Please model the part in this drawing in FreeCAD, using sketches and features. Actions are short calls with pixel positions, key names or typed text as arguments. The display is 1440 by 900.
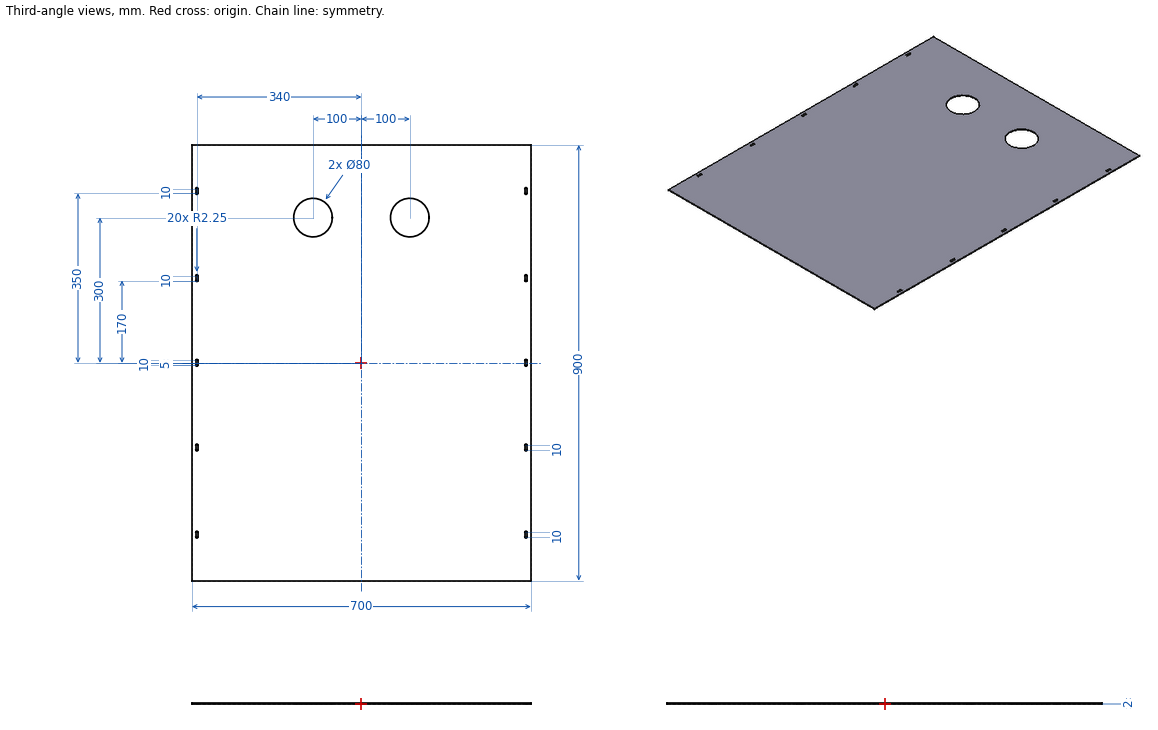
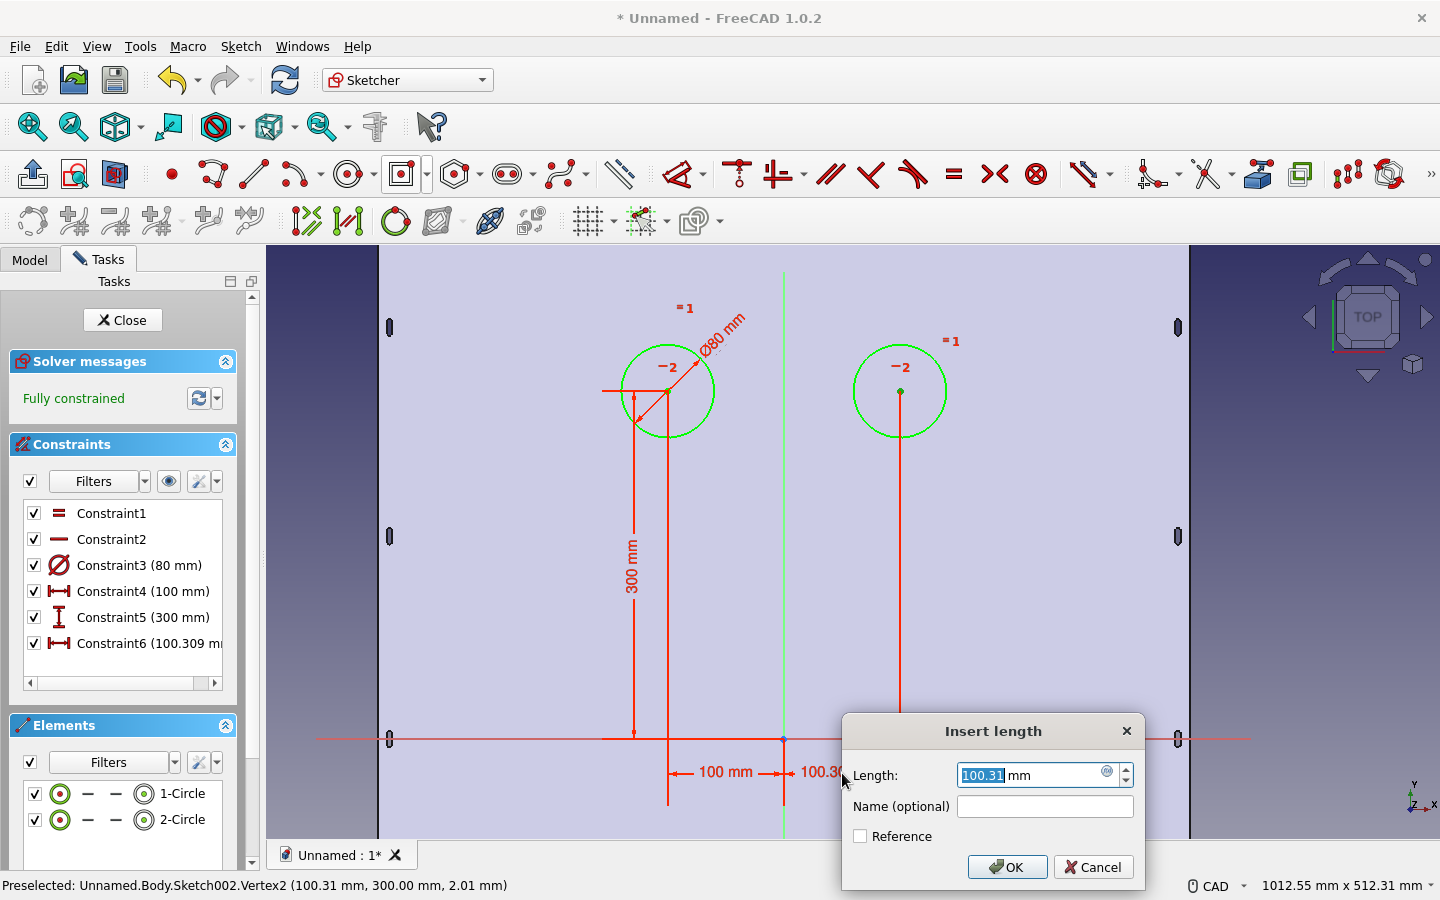
text(100)
key(Return)
key(Escape)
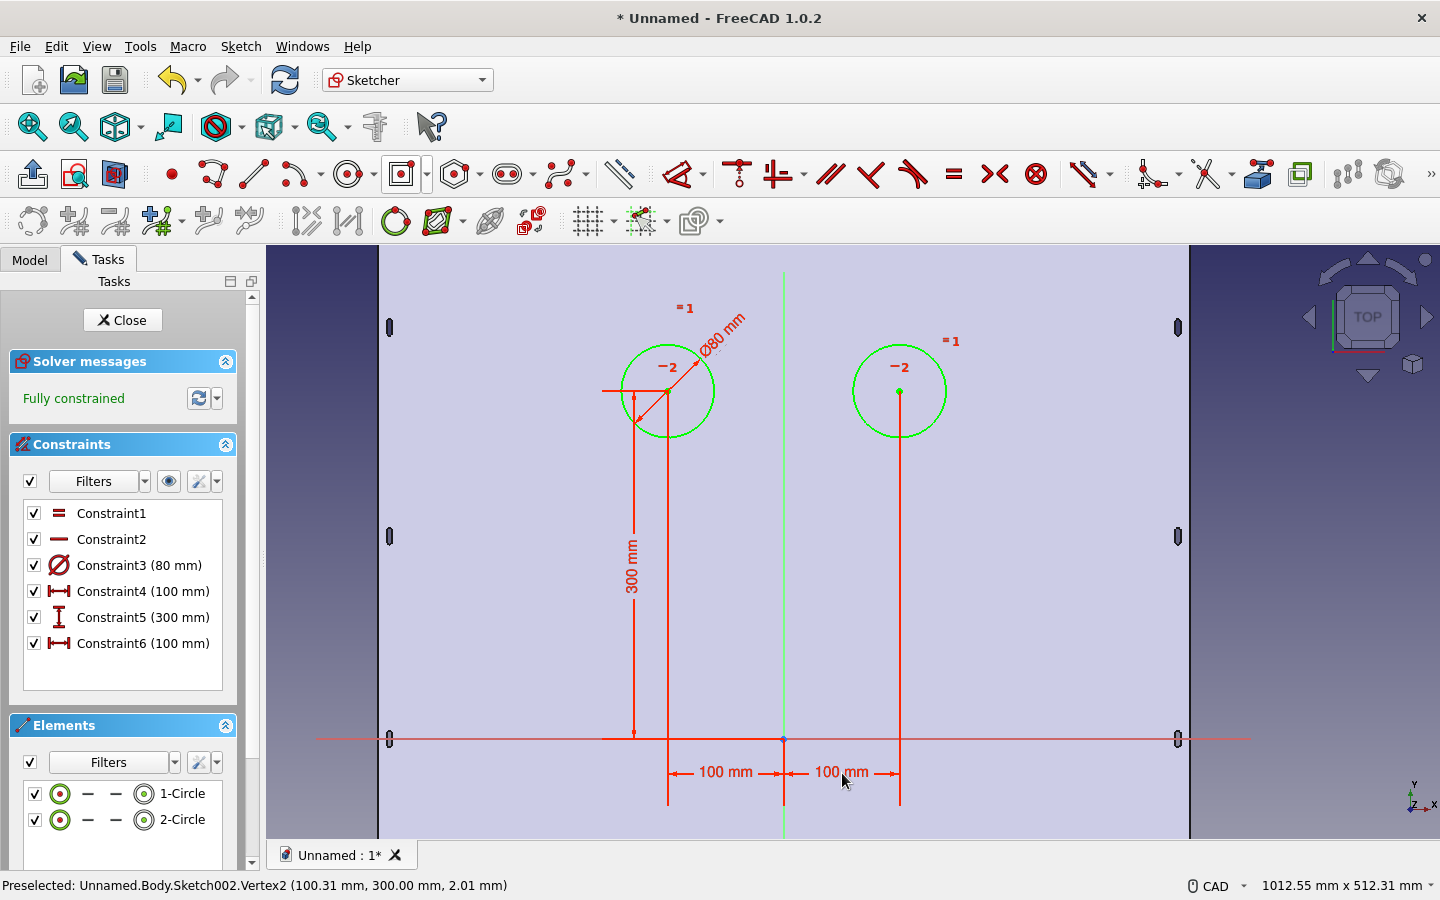
click(123, 320)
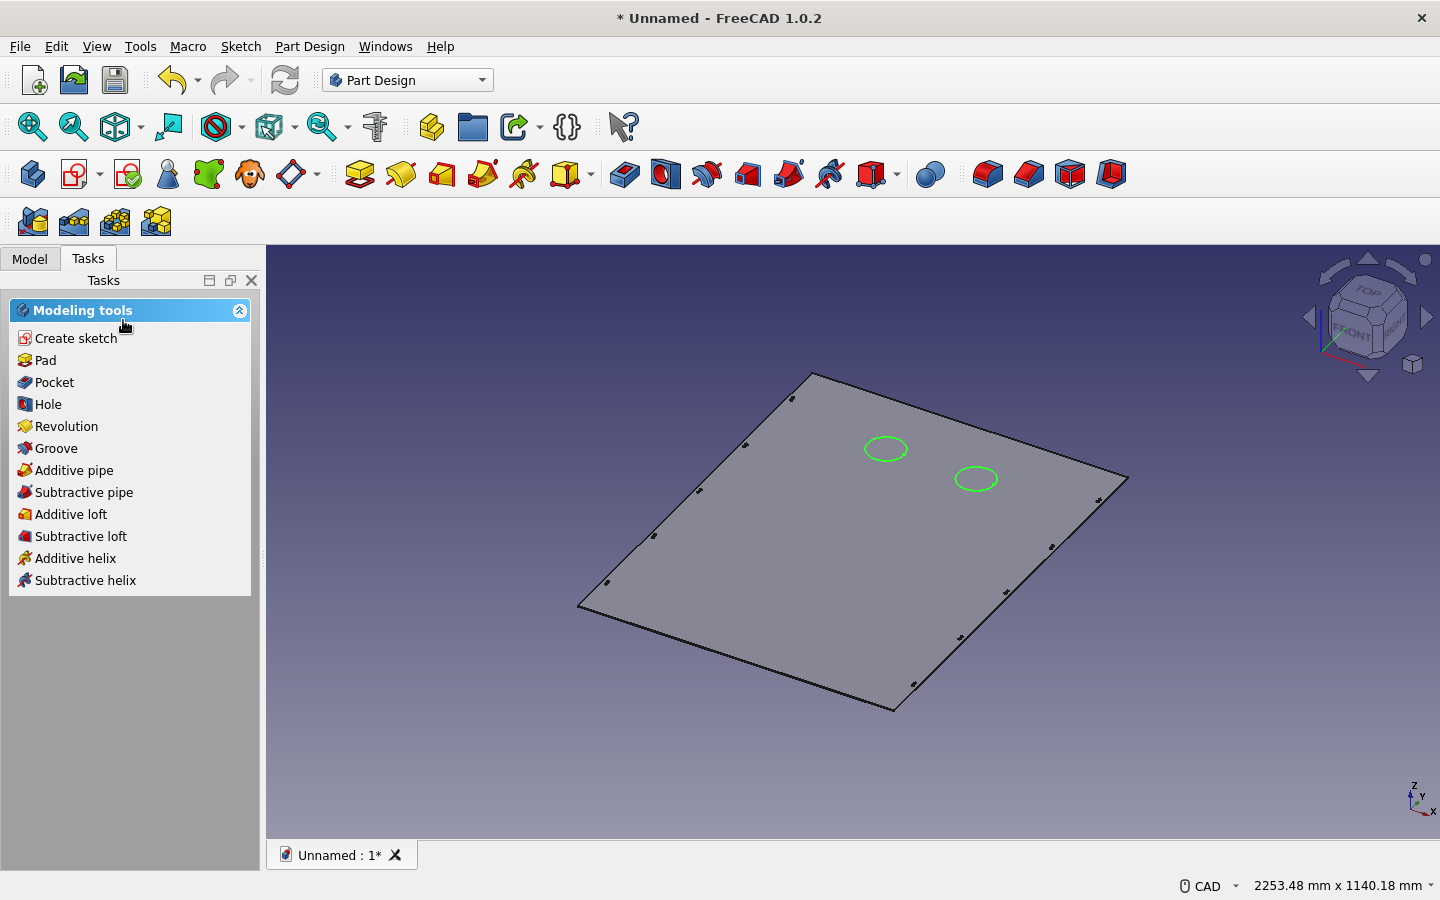
click(625, 174)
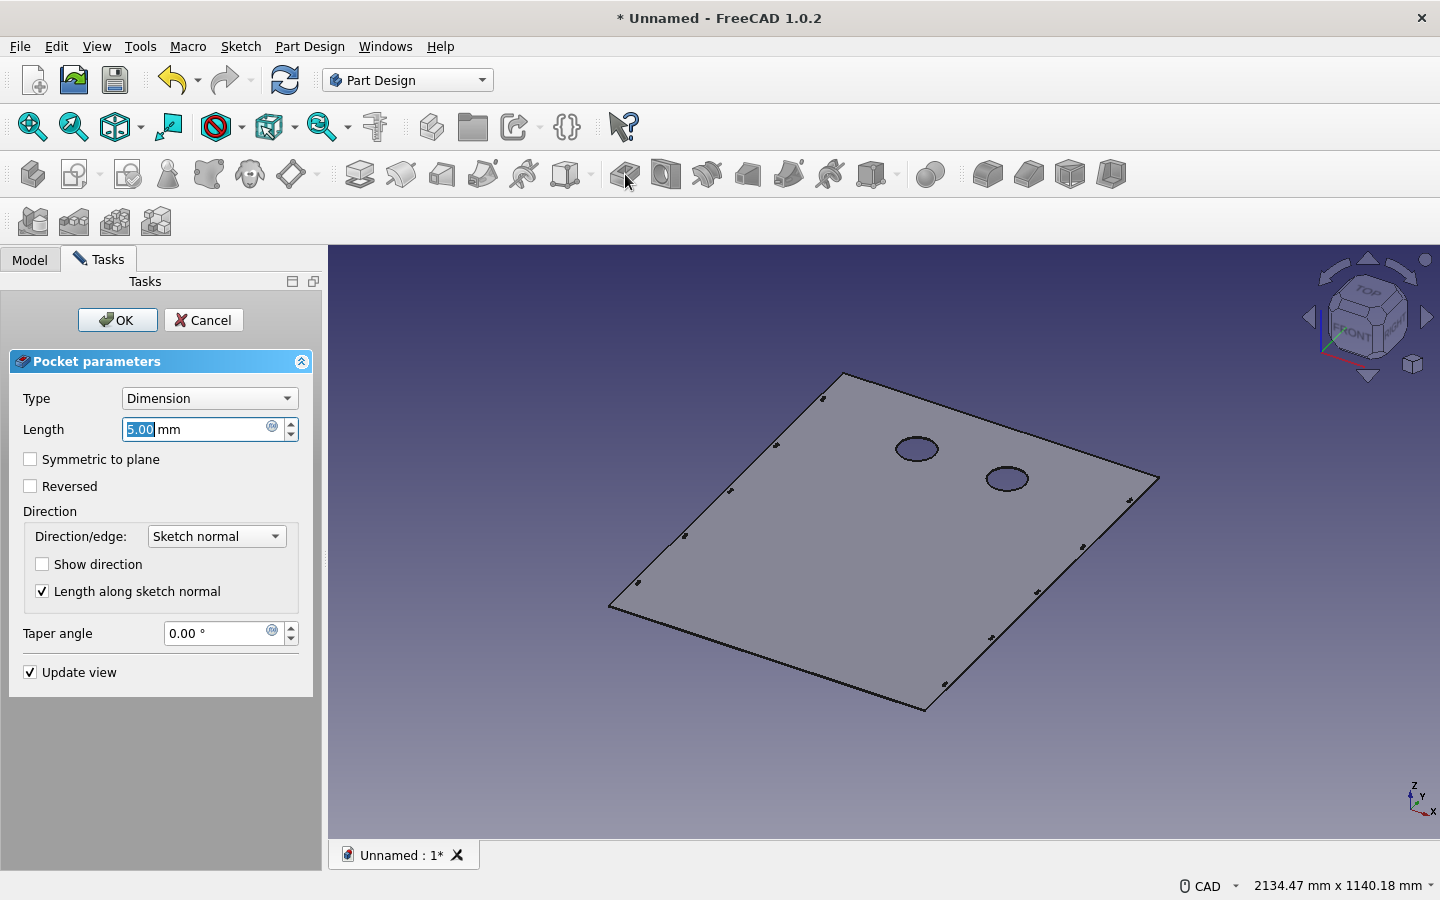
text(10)
key(Tab)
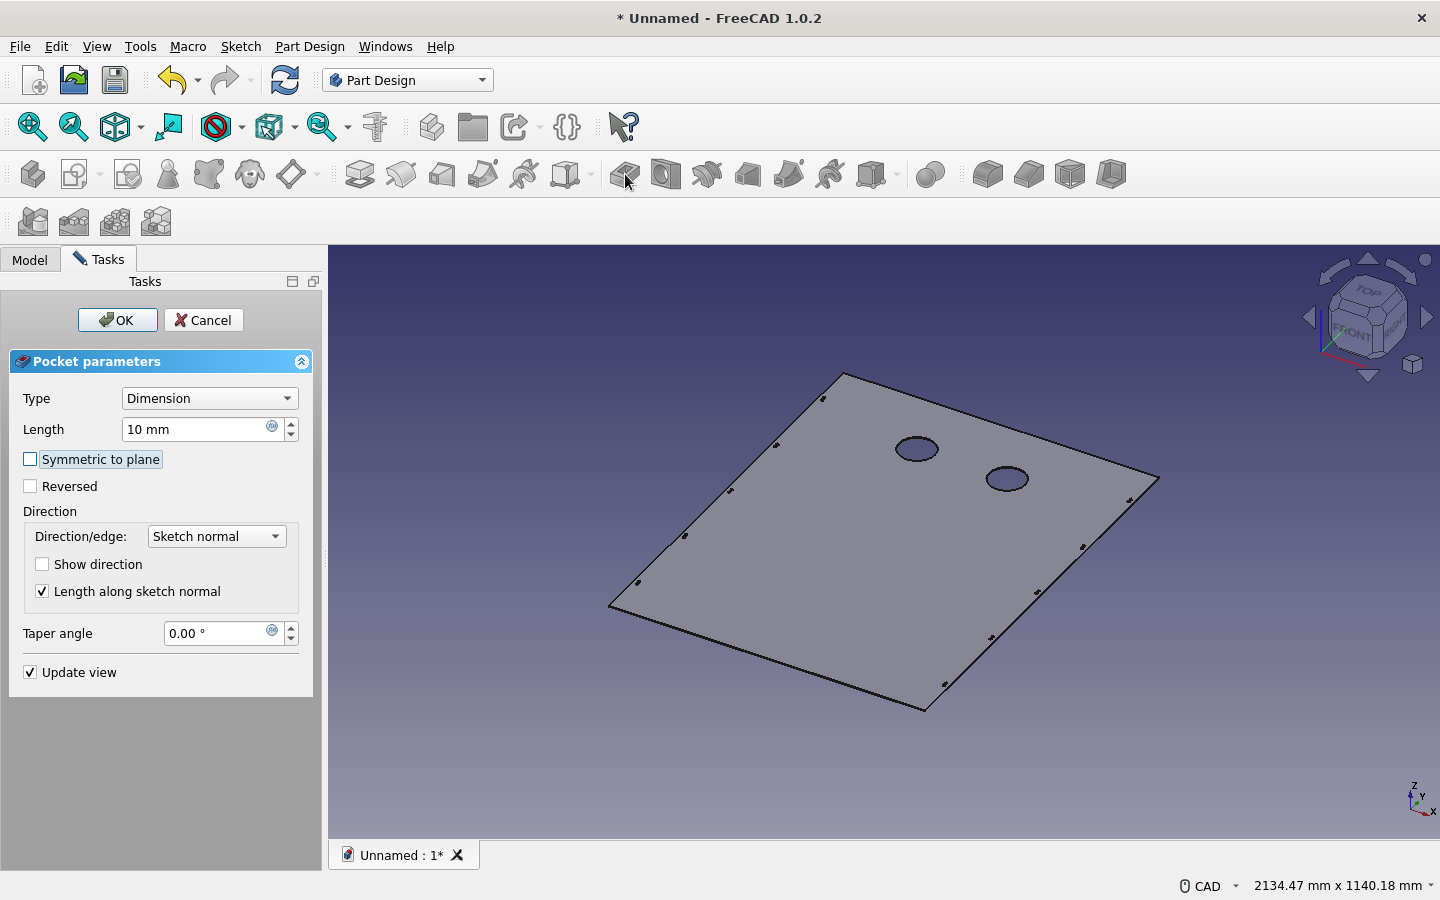
click(118, 320)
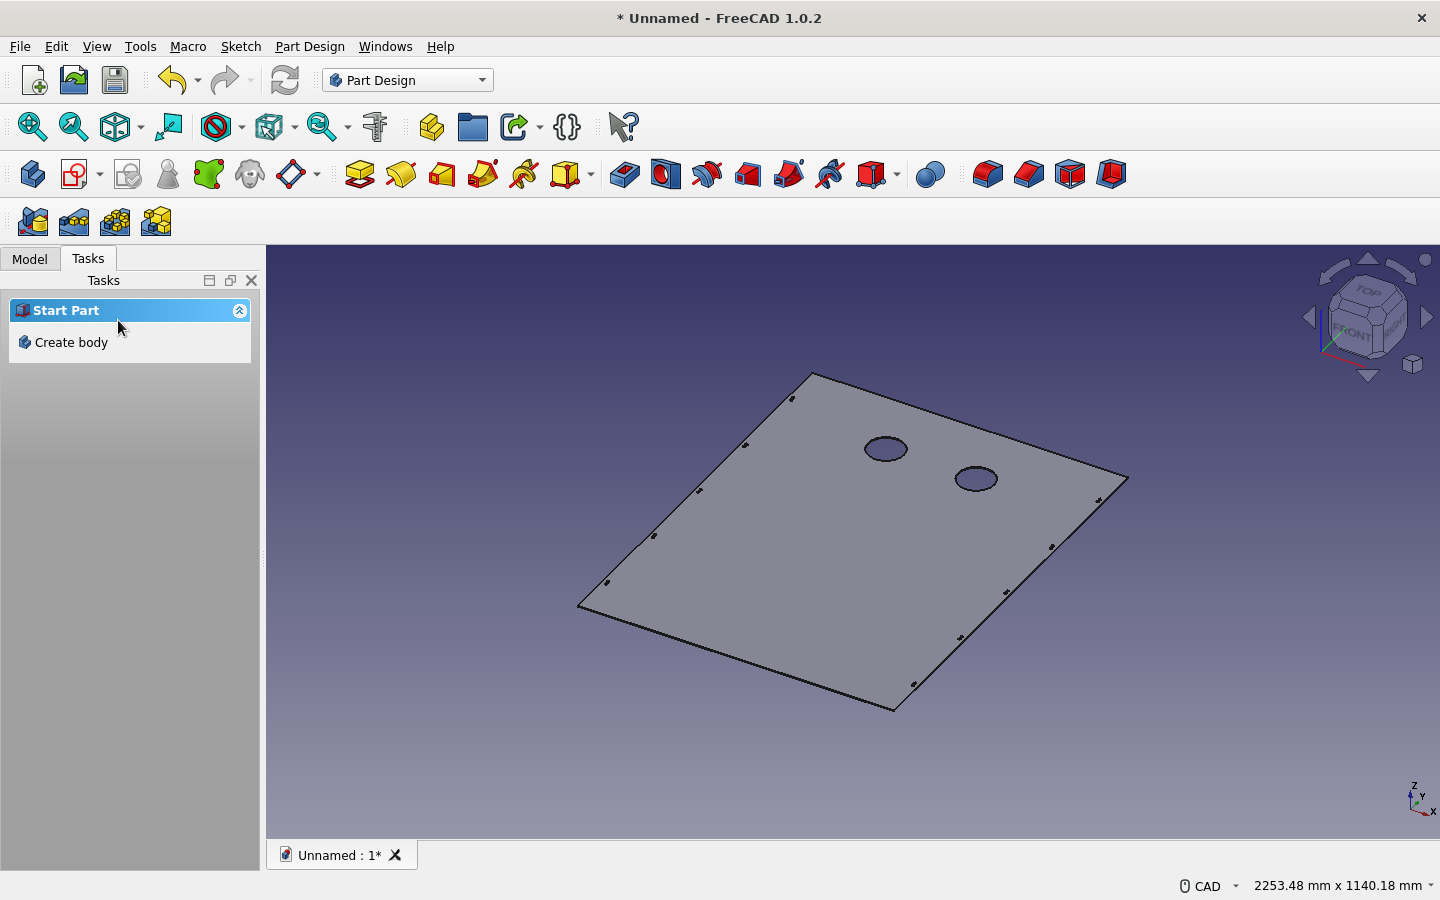
key(0)